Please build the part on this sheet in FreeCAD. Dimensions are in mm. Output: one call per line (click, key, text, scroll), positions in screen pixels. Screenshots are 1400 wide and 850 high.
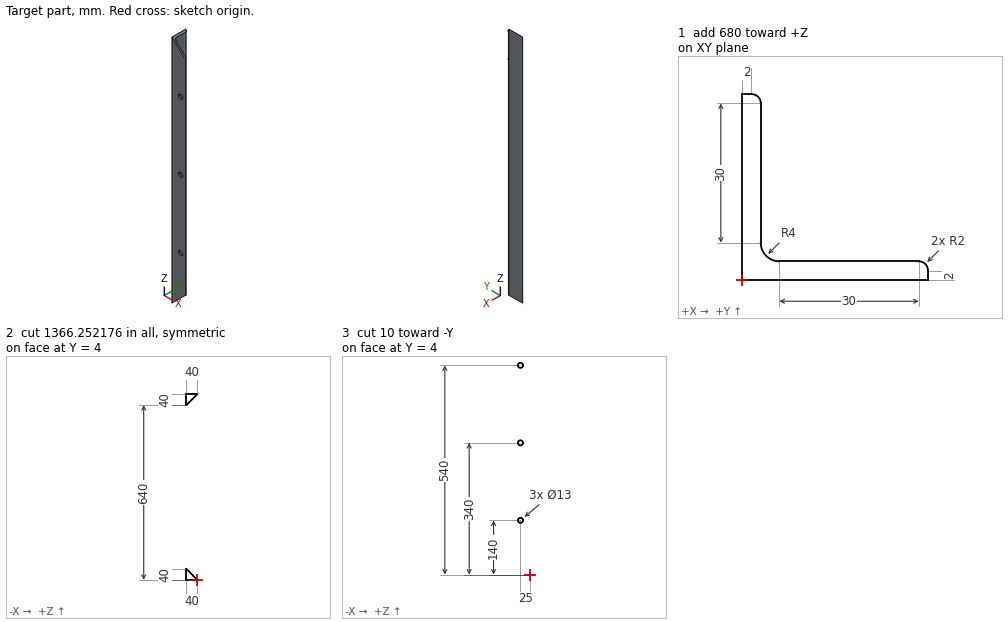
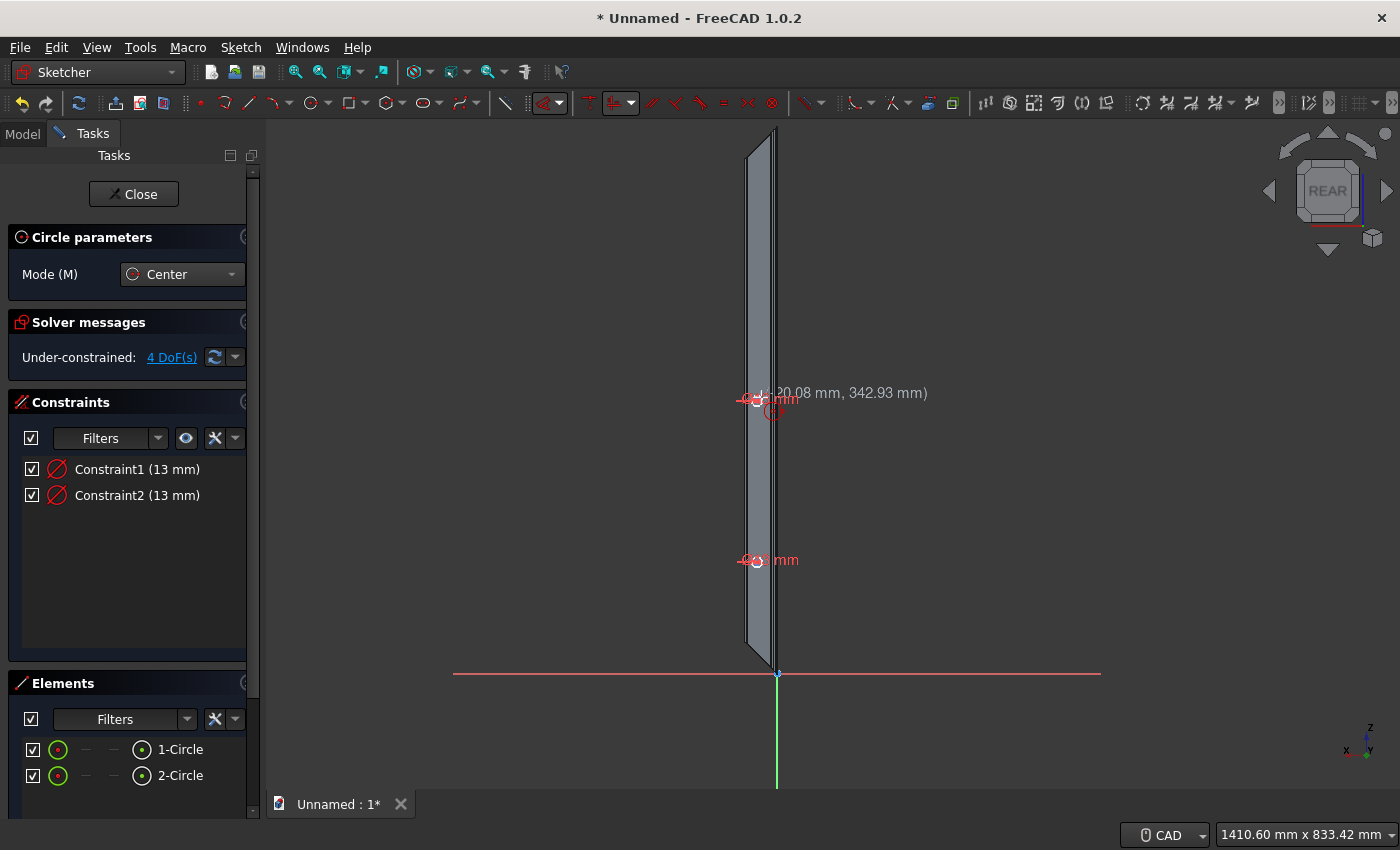
scroll(757, 240, up, 8)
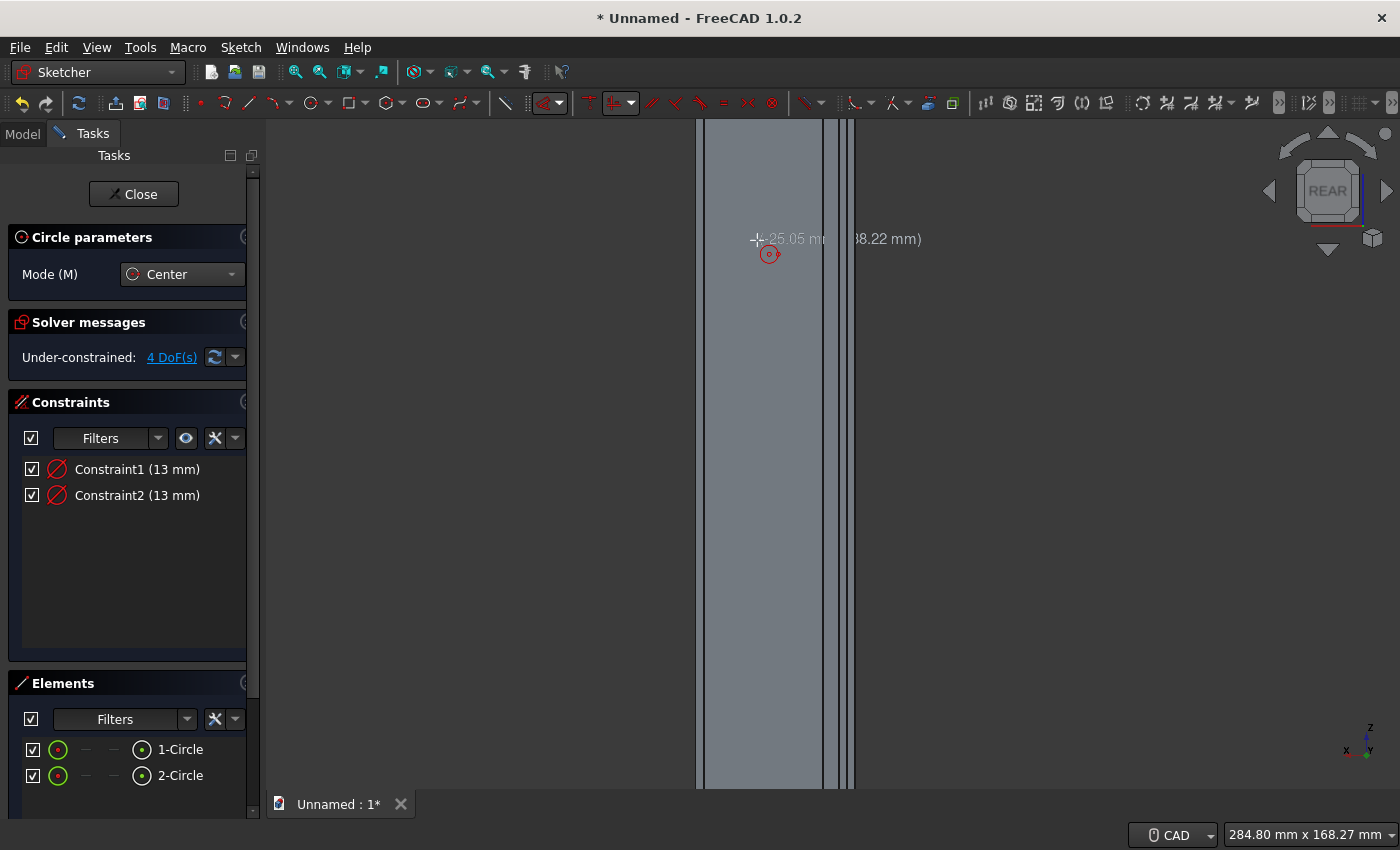
scroll(757, 240, down, 8)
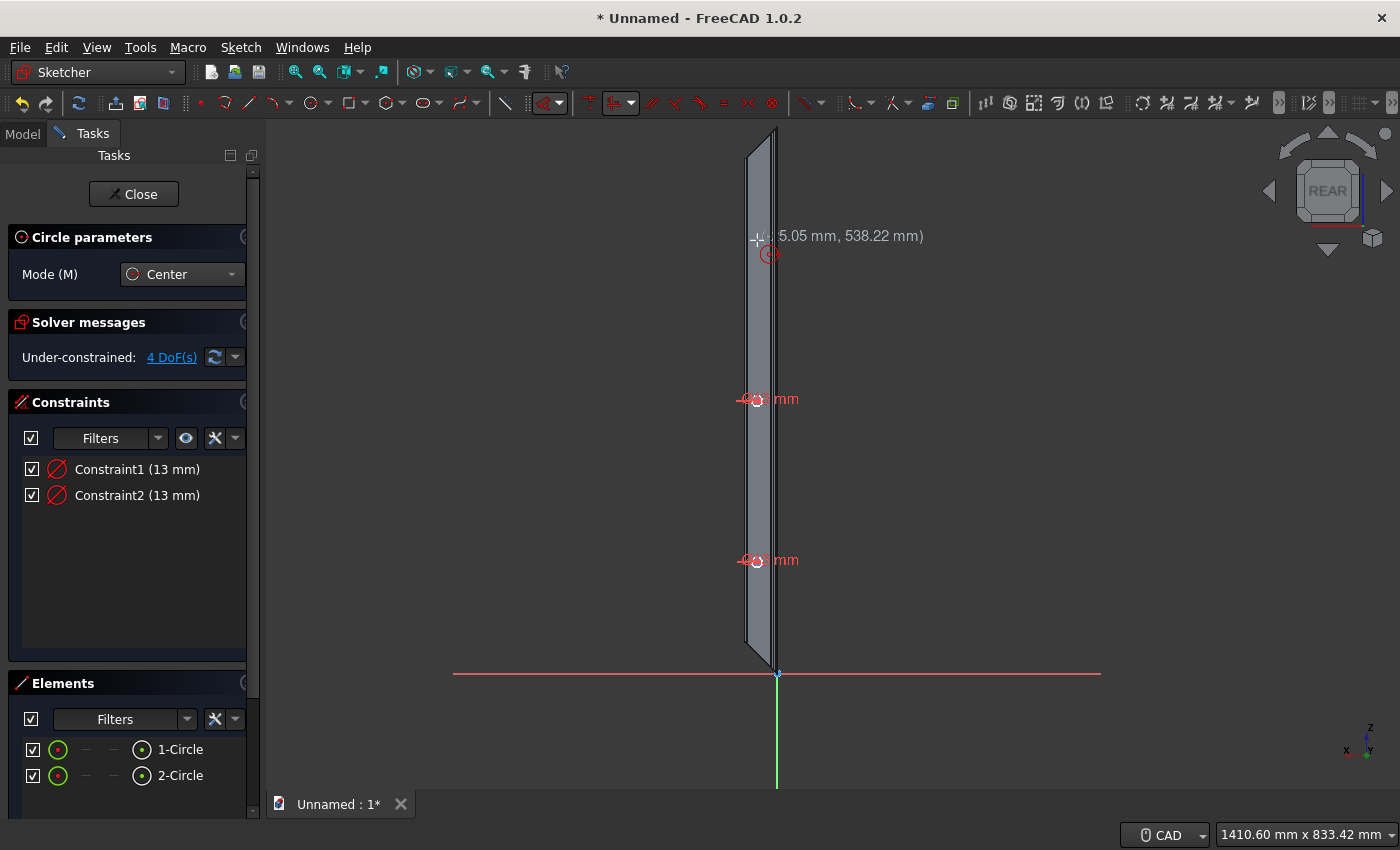
click(757, 240)
move(761, 236)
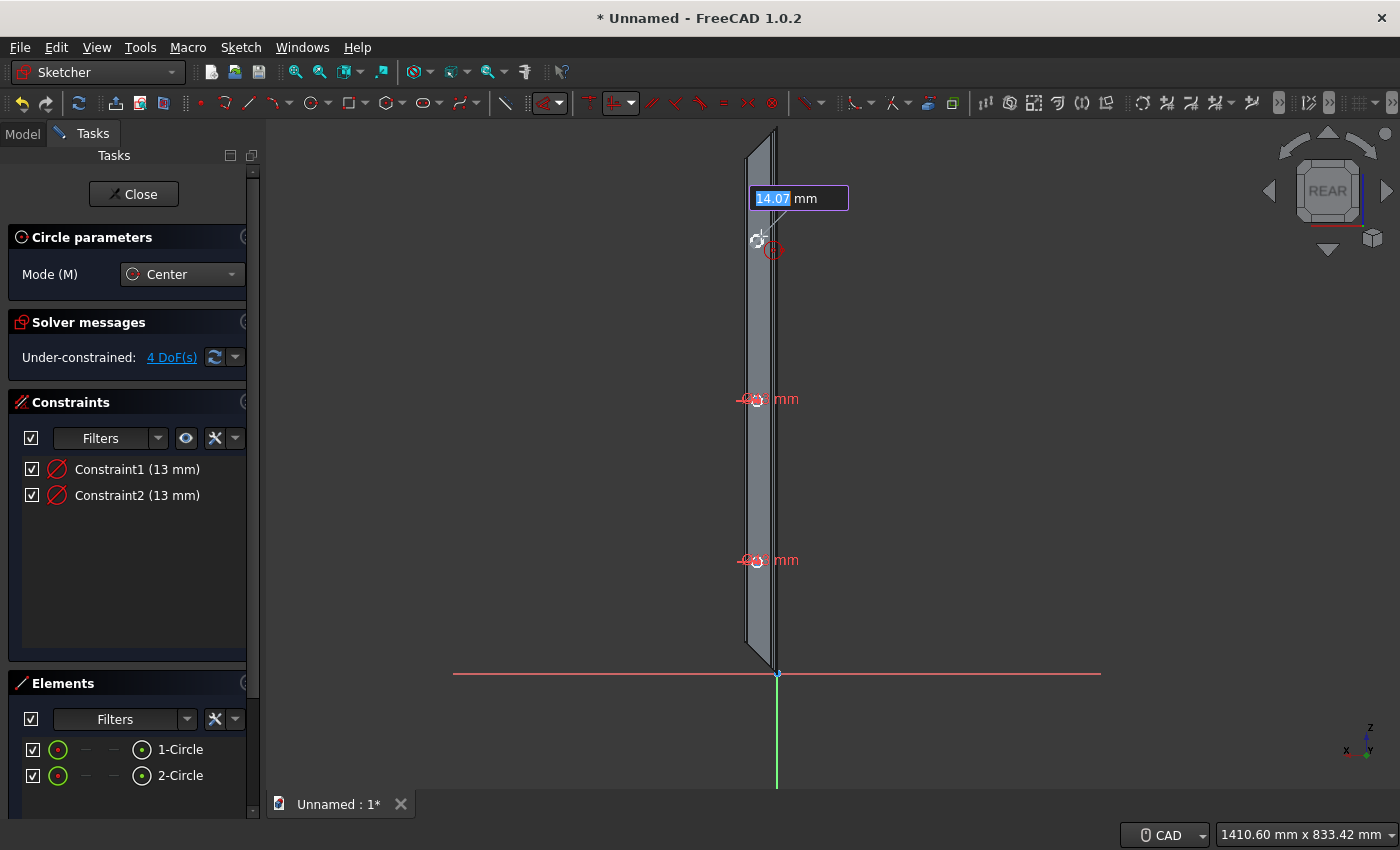
text(13)
key(Return)
key(Escape)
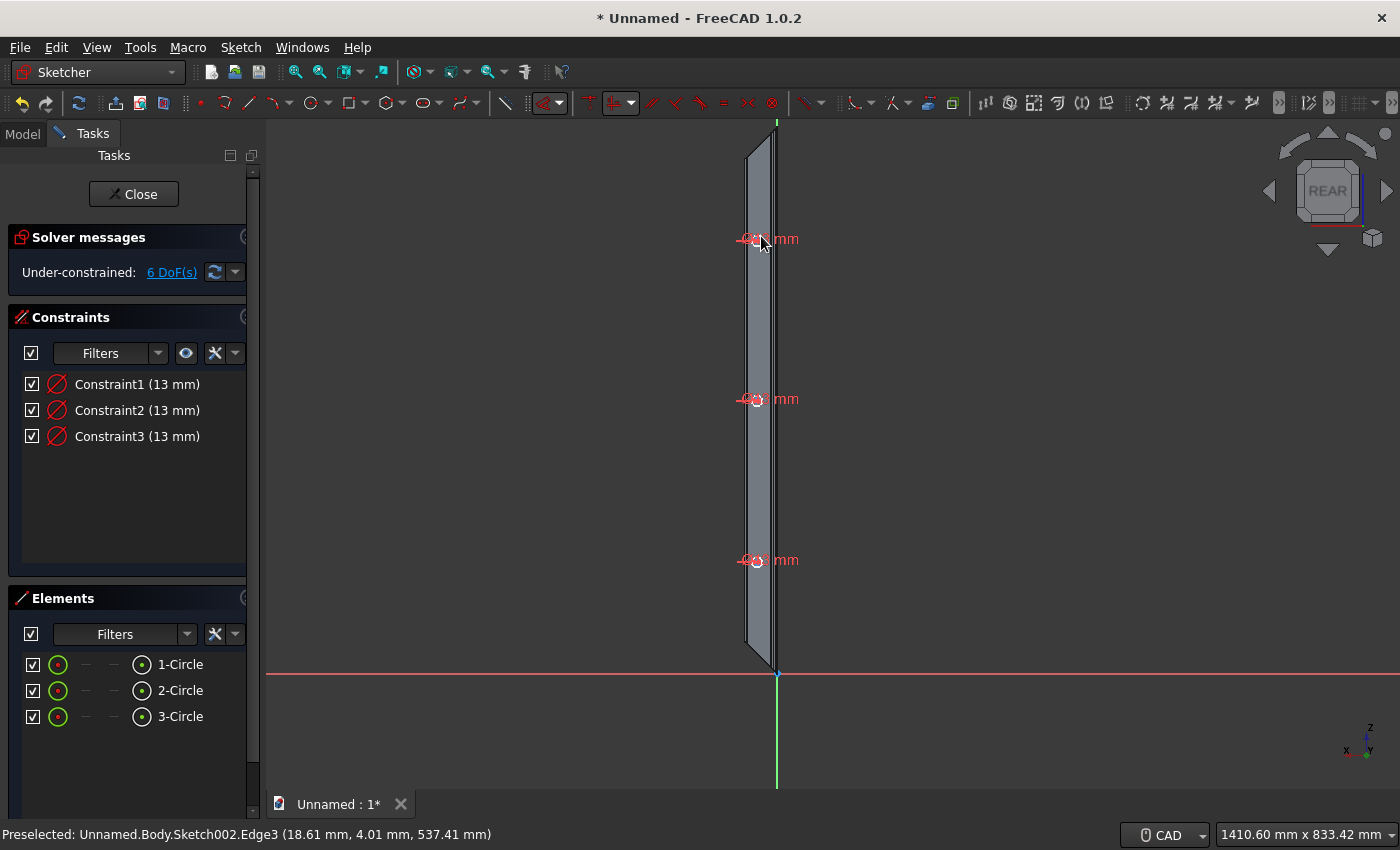
click(757, 562)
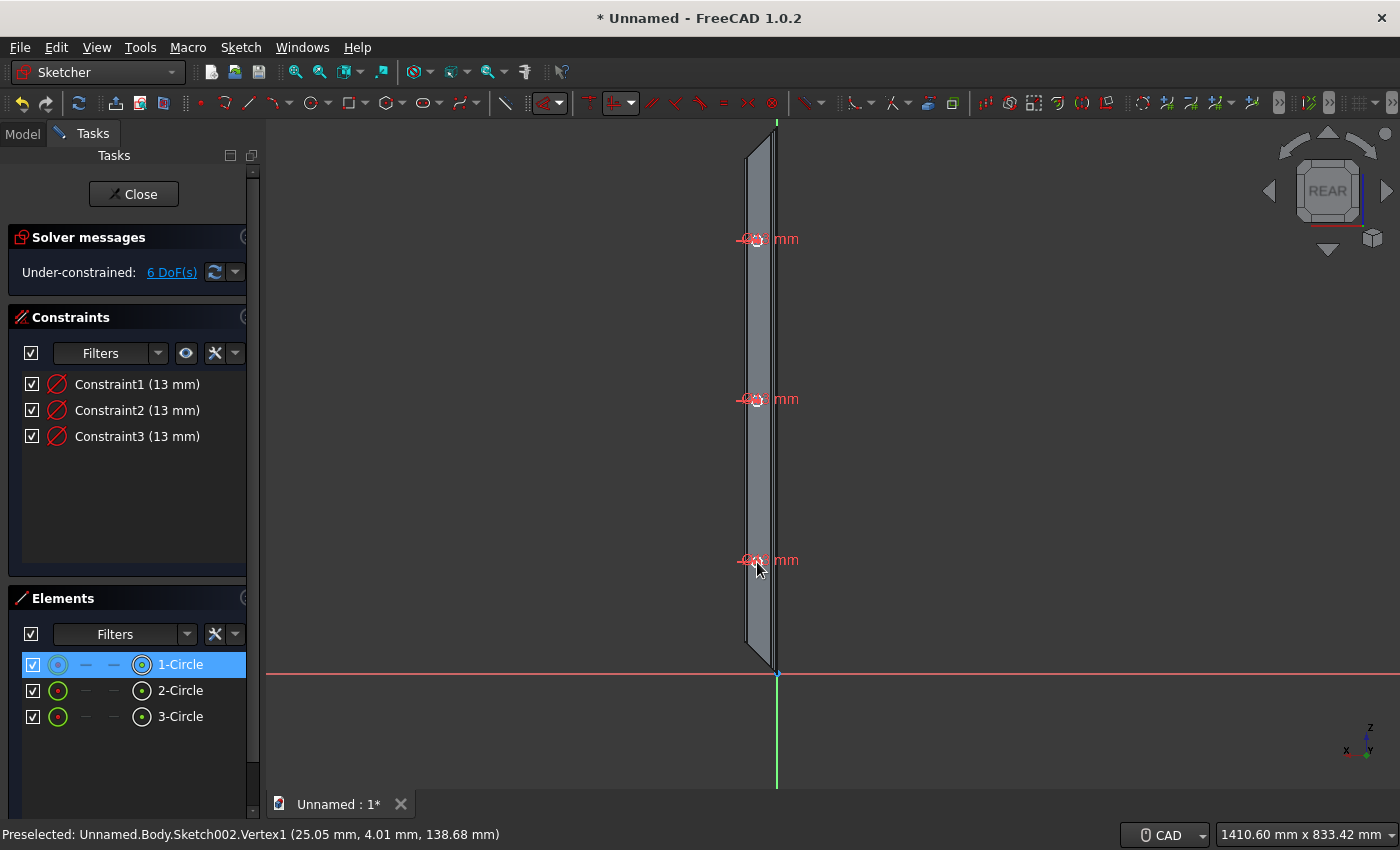
click(757, 401)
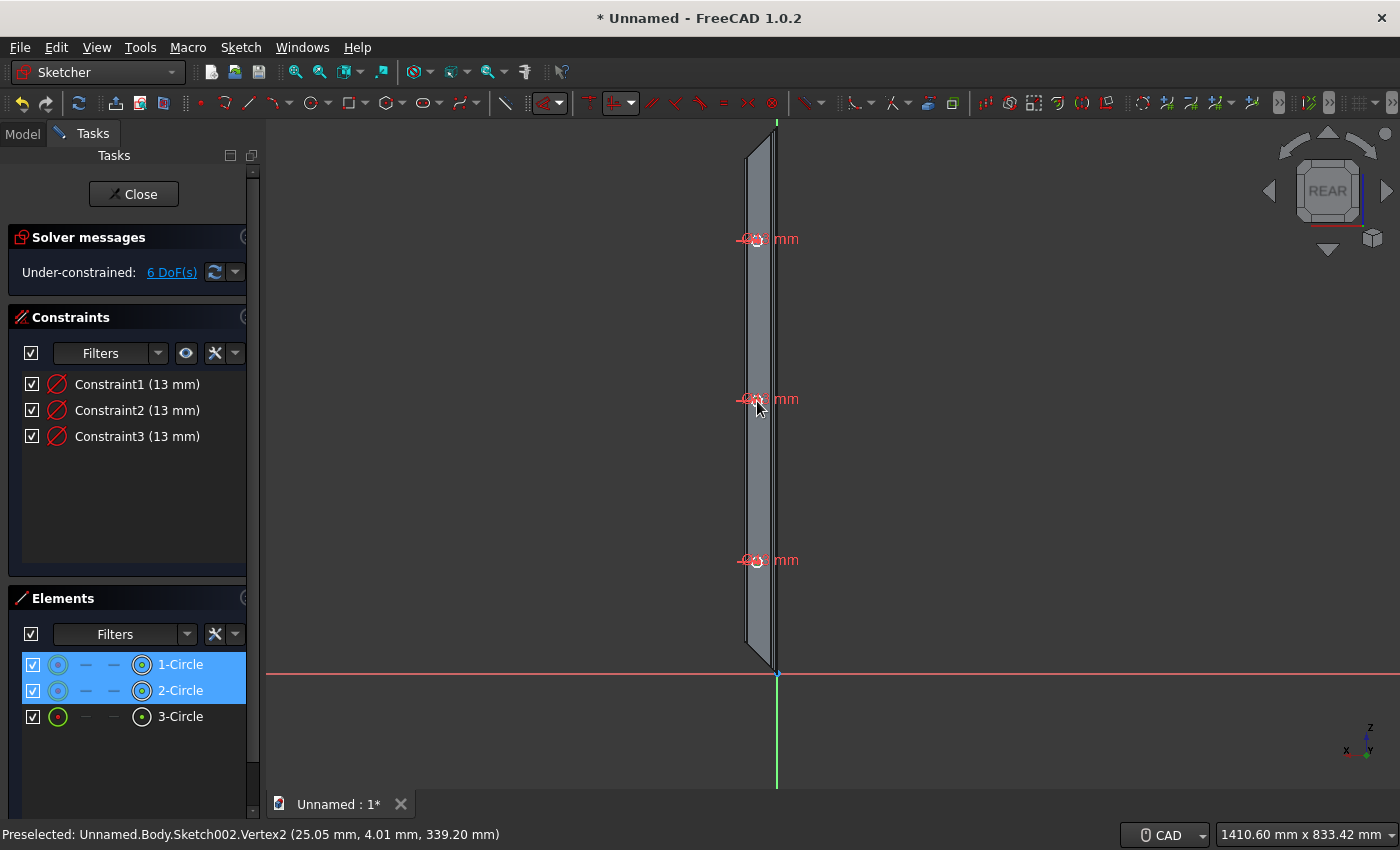
key(v)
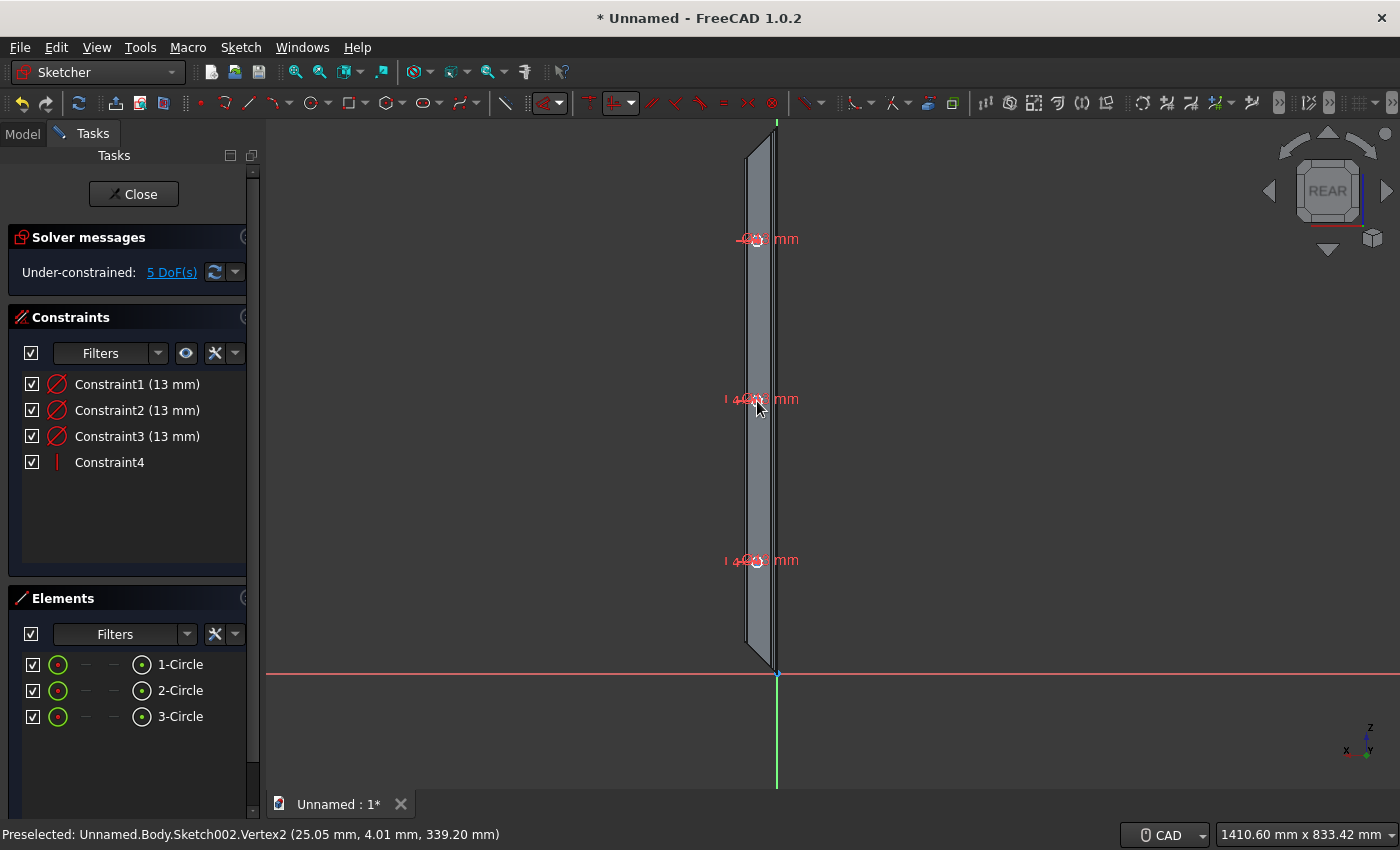
click(757, 401)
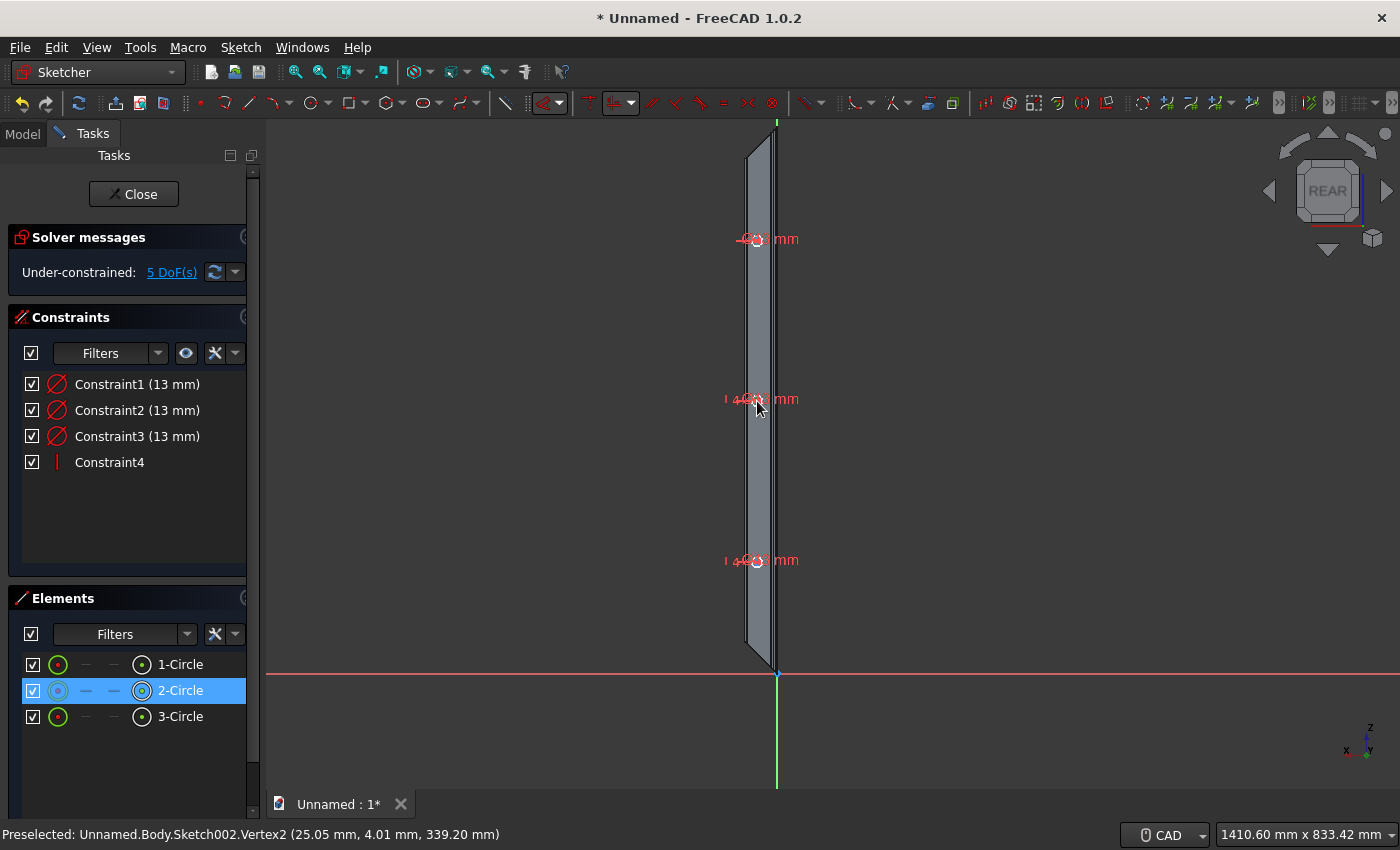
click(757, 241)